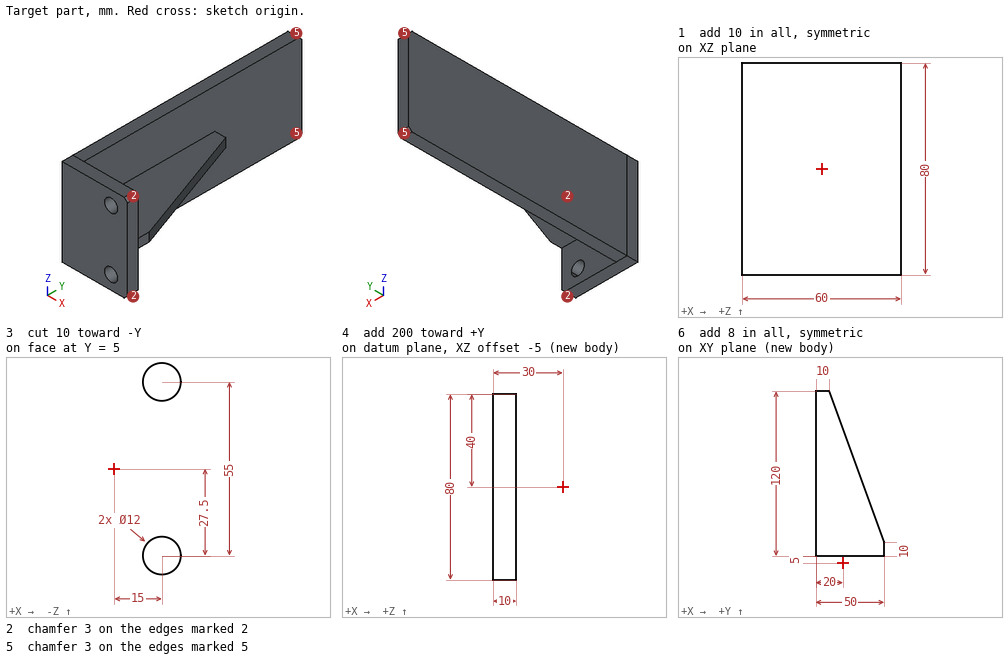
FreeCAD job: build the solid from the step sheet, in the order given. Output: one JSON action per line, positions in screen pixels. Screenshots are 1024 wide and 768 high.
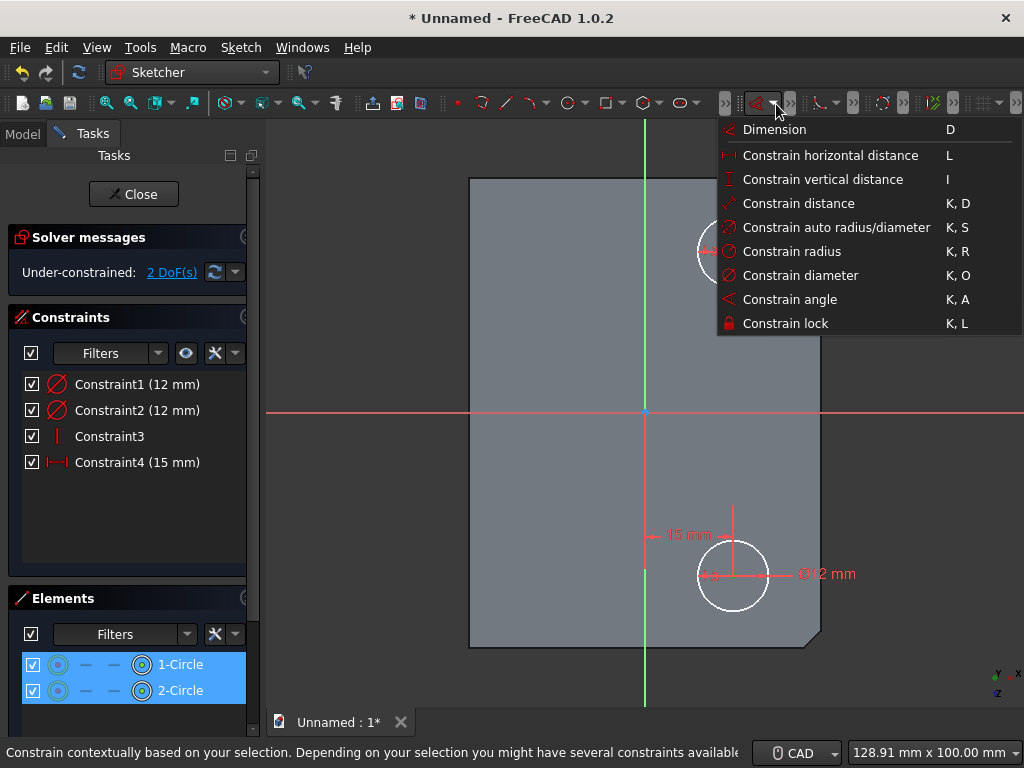
{"action": "left_click", "coordinate": [870, 179]}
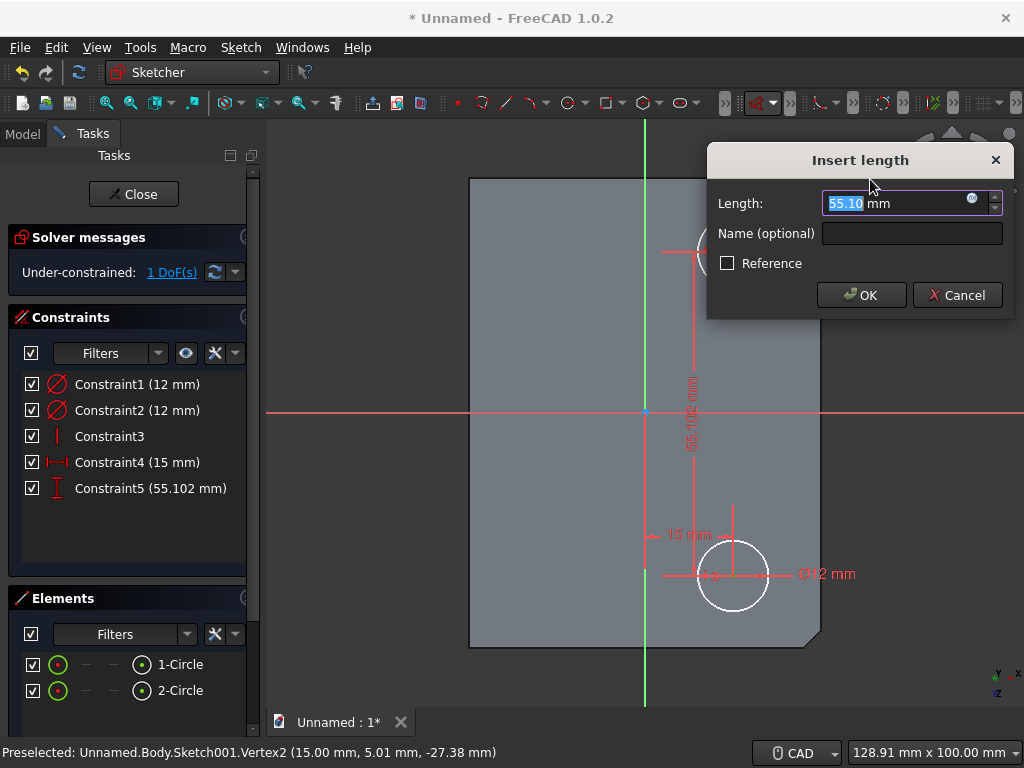
{"action": "type", "text": "55"}
{"action": "key", "text": "Return"}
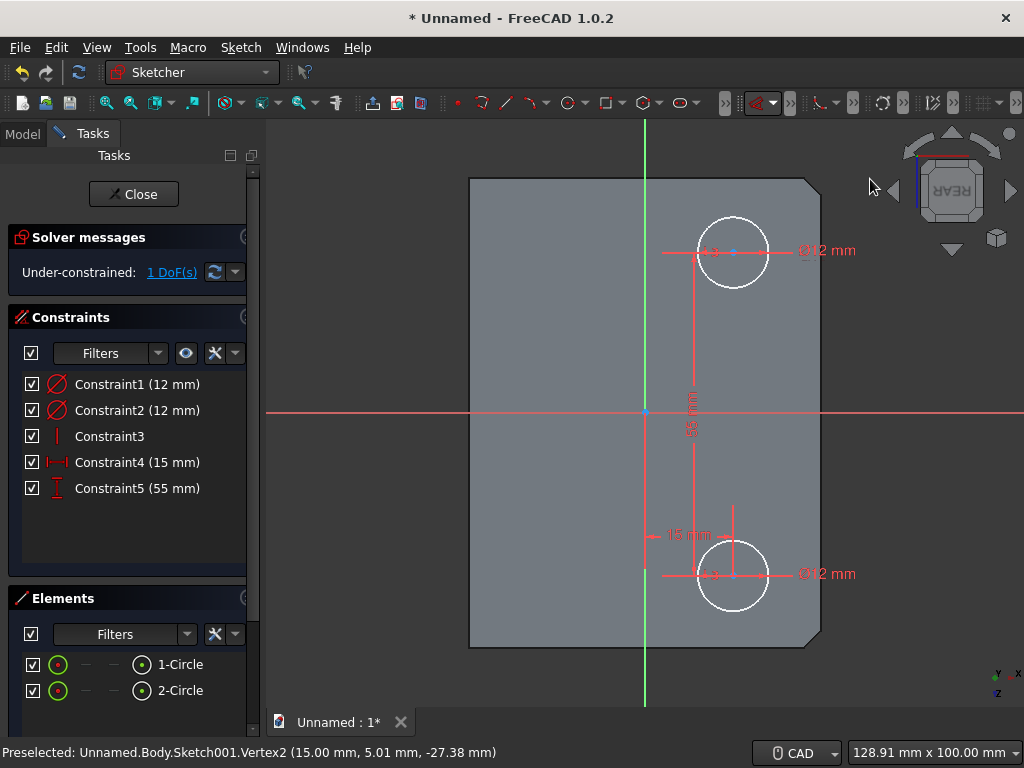
{"action": "left_click", "coordinate": [733, 576]}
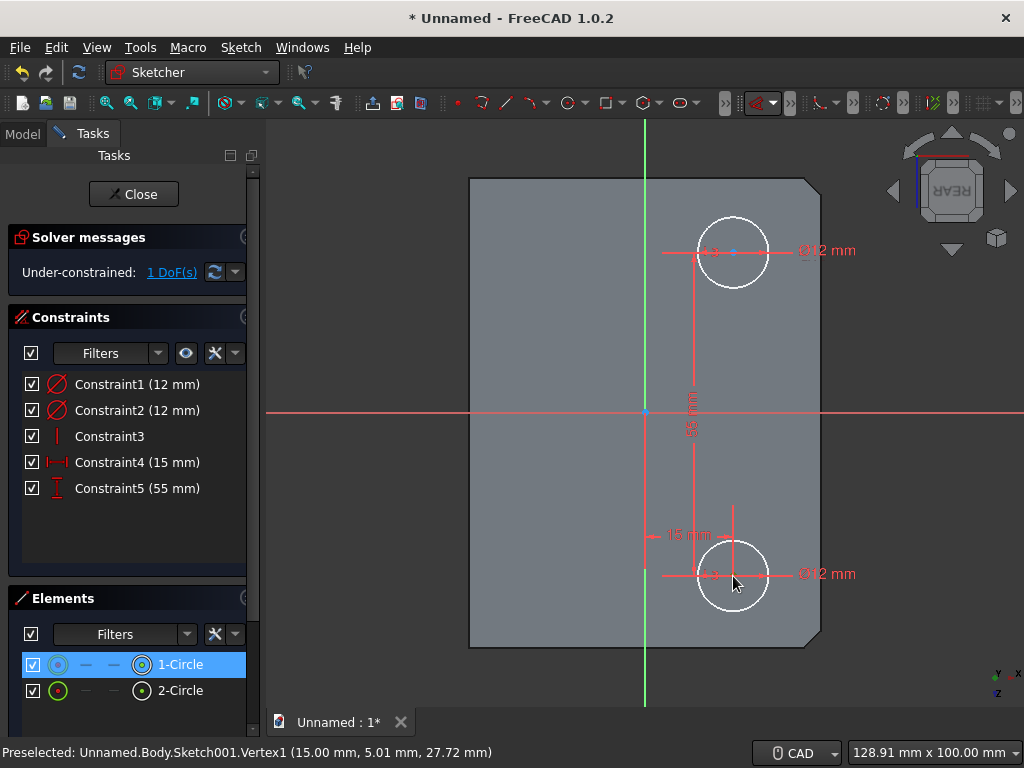
{"action": "key", "text": "i"}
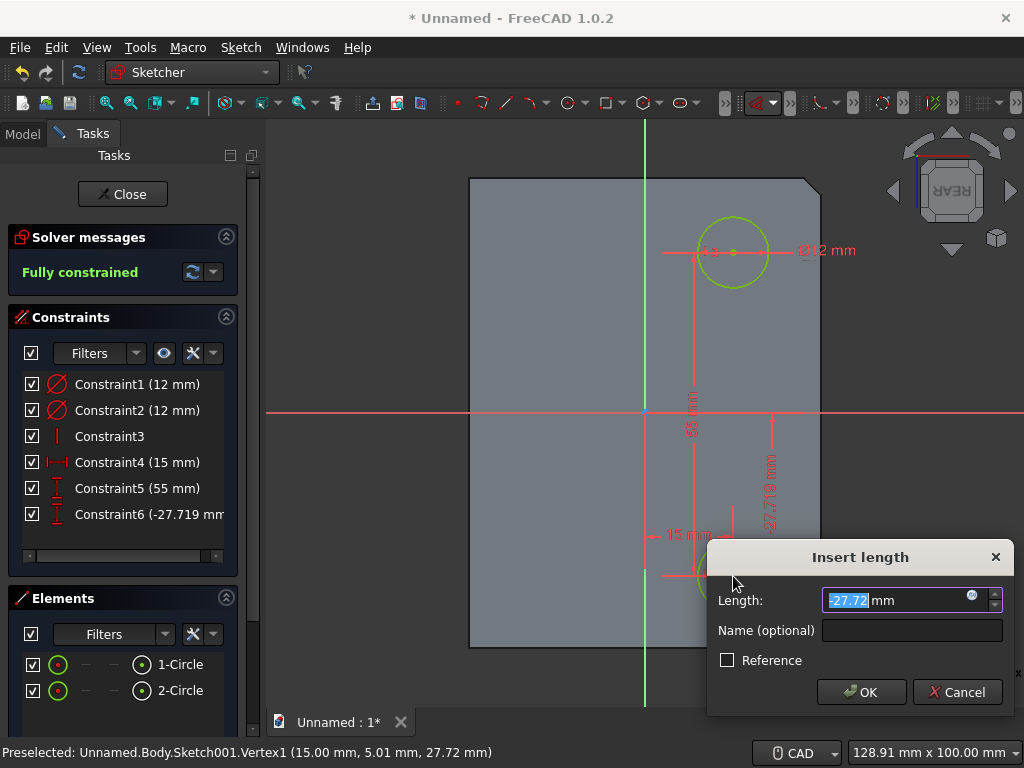
{"action": "type", "text": "-27.5"}
{"action": "key", "text": "Return"}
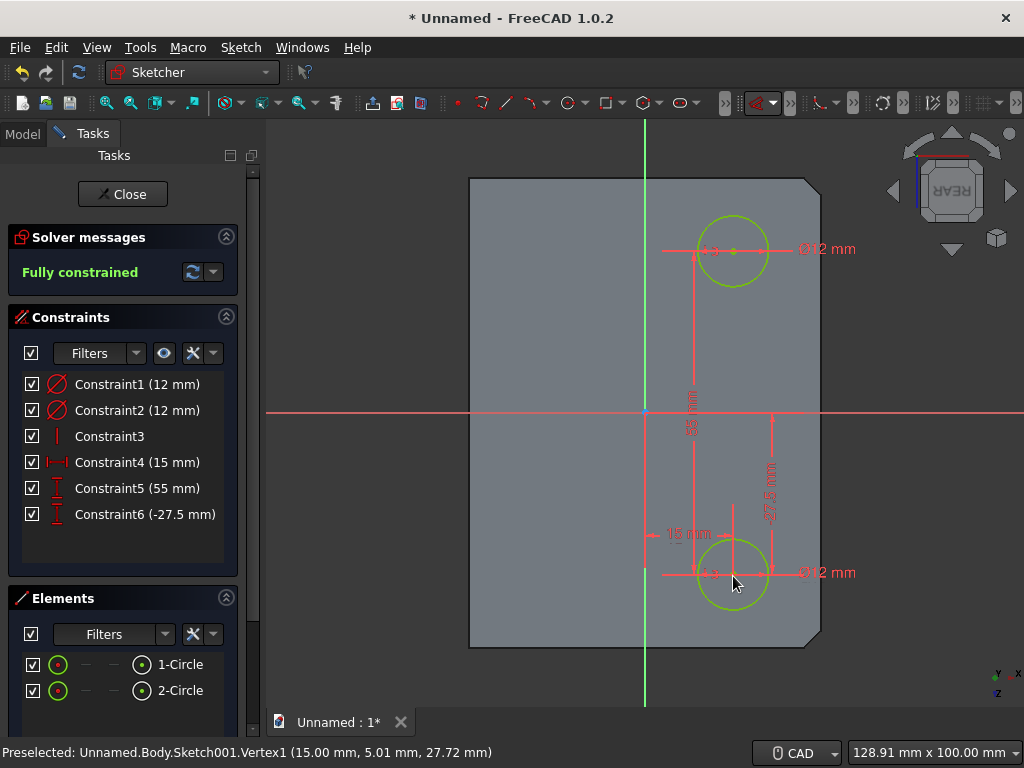
{"action": "left_click", "coordinate": [123, 194]}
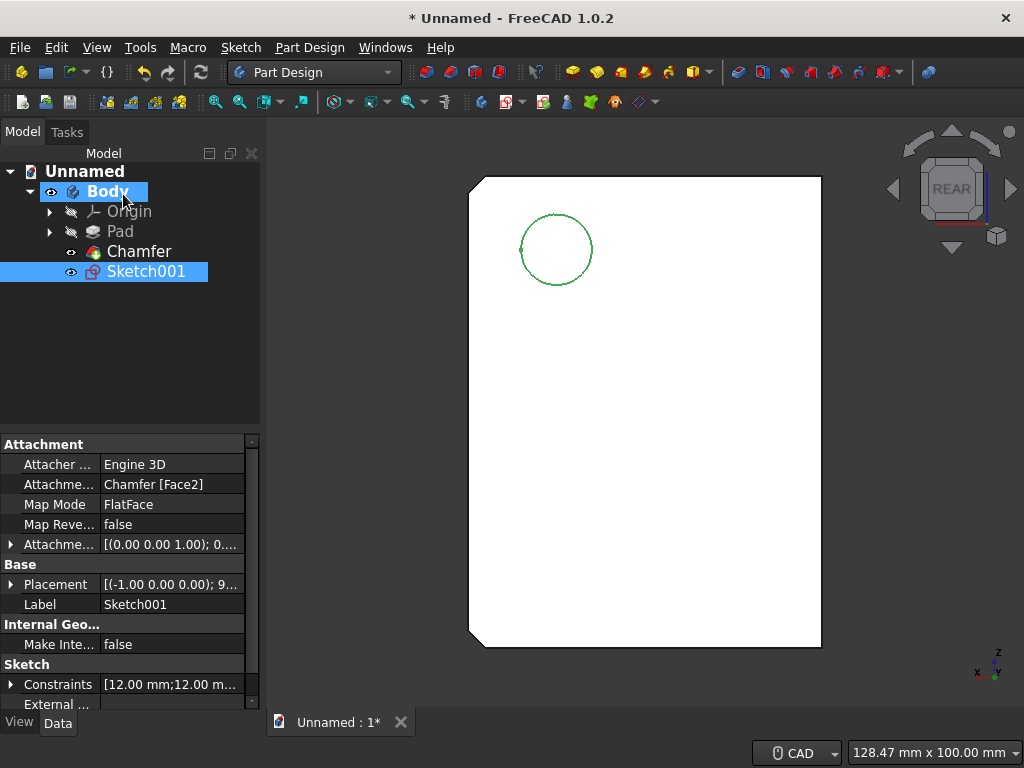
{"action": "left_click", "coordinate": [740, 72]}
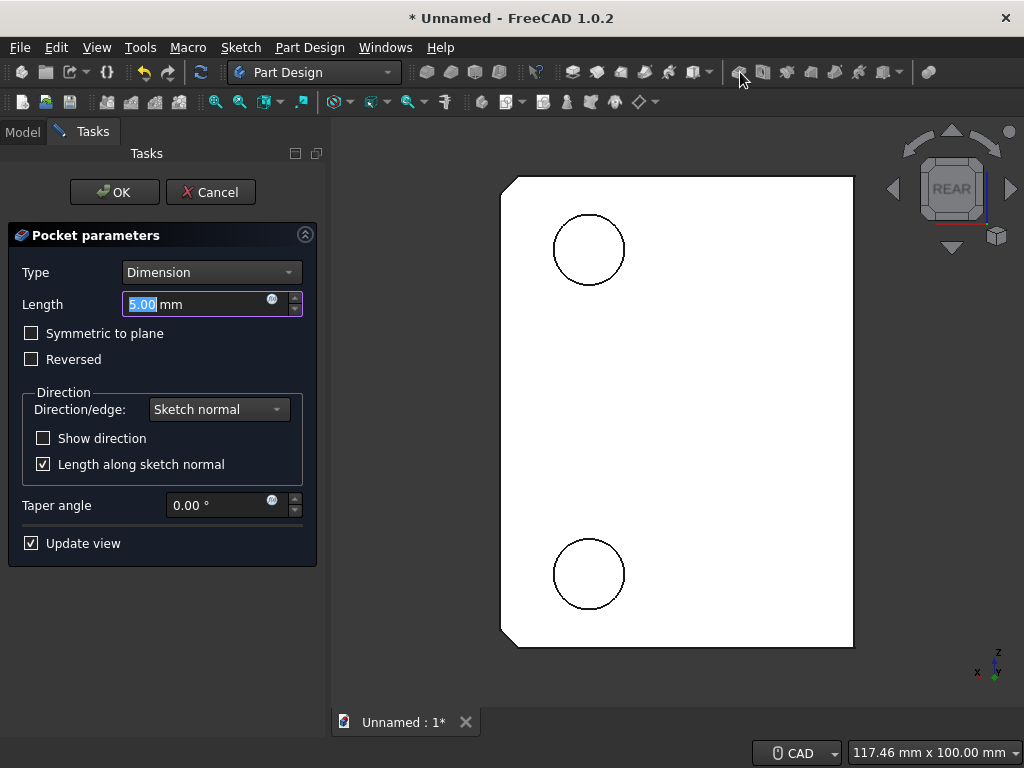
{"action": "type", "text": "10"}
{"action": "key", "text": "Tab"}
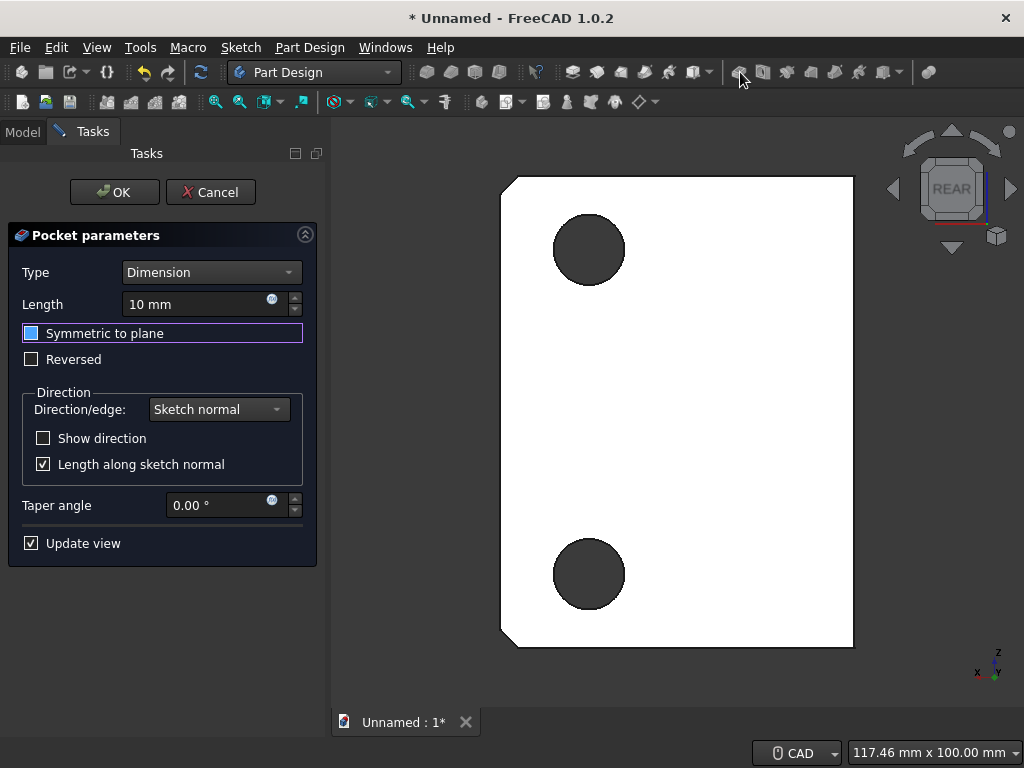
{"action": "left_click", "coordinate": [115, 192]}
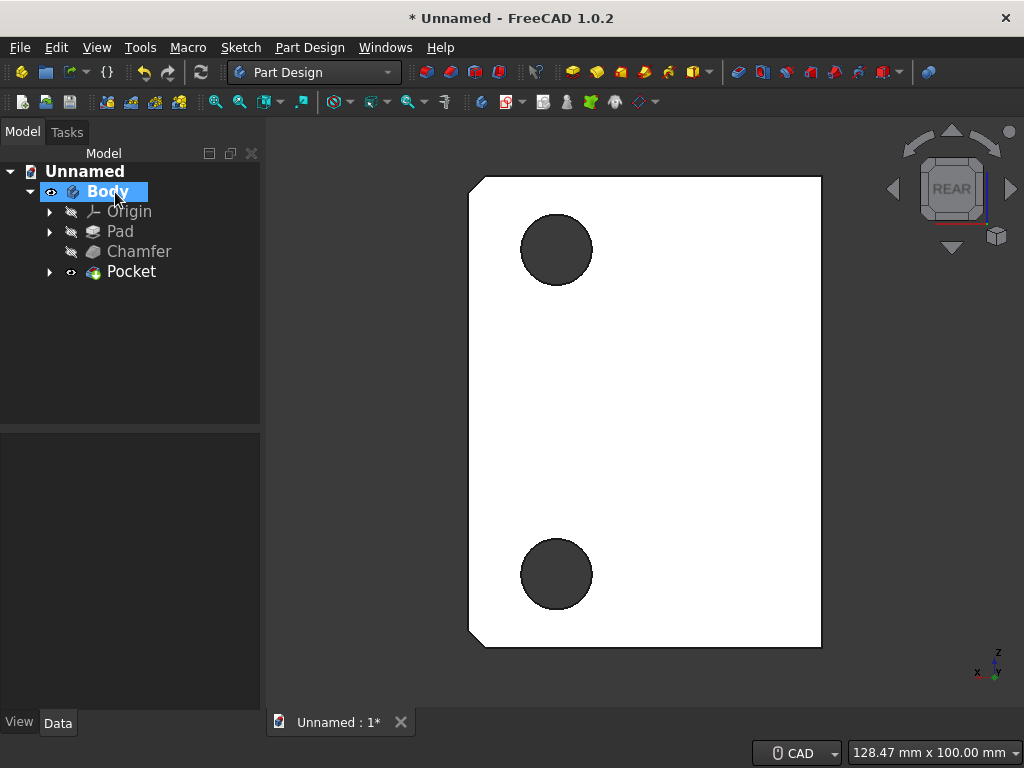
{"action": "left_click", "coordinate": [482, 102]}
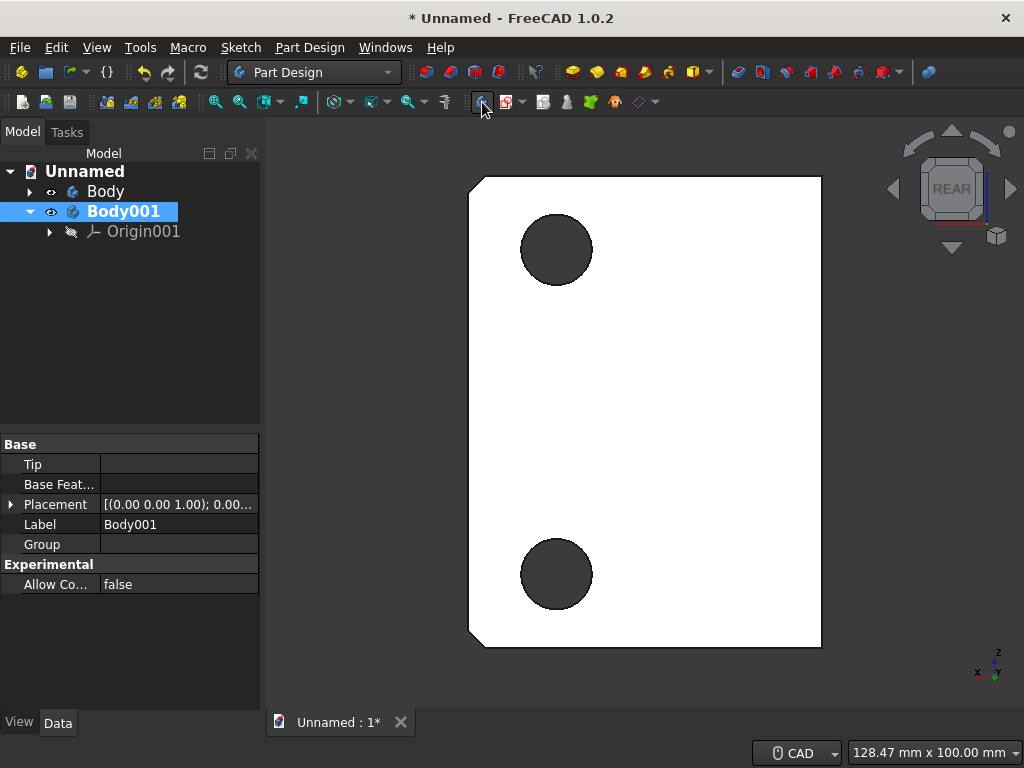
{"action": "left_click", "coordinate": [50, 232]}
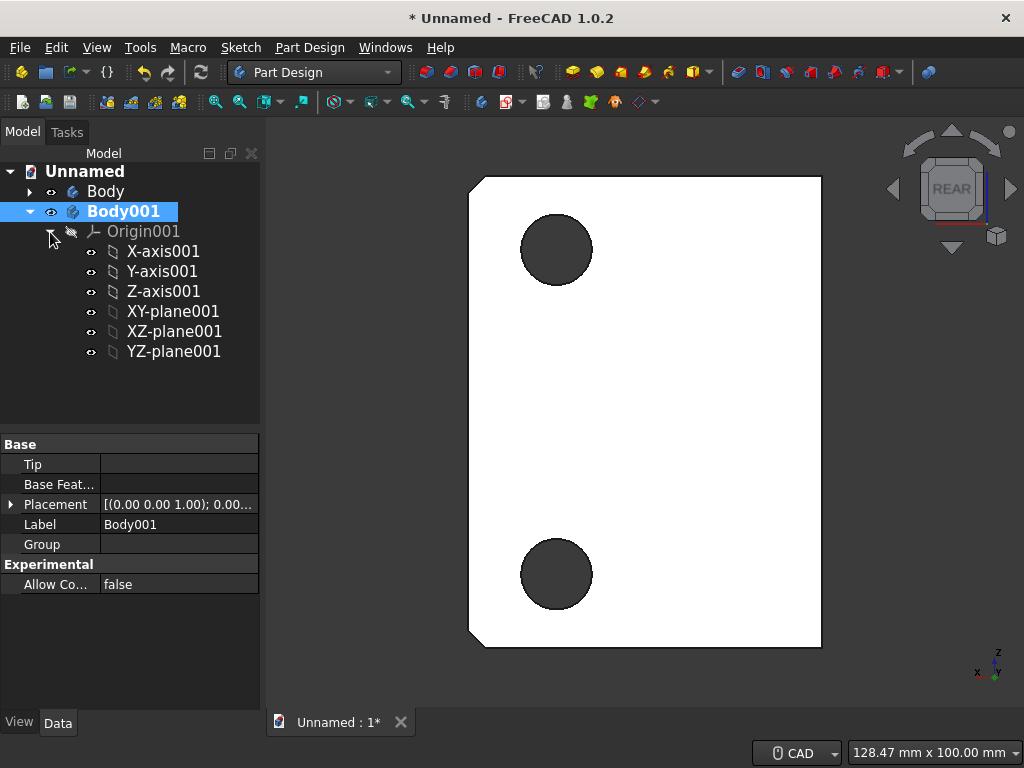
{"action": "left_click", "coordinate": [136, 332]}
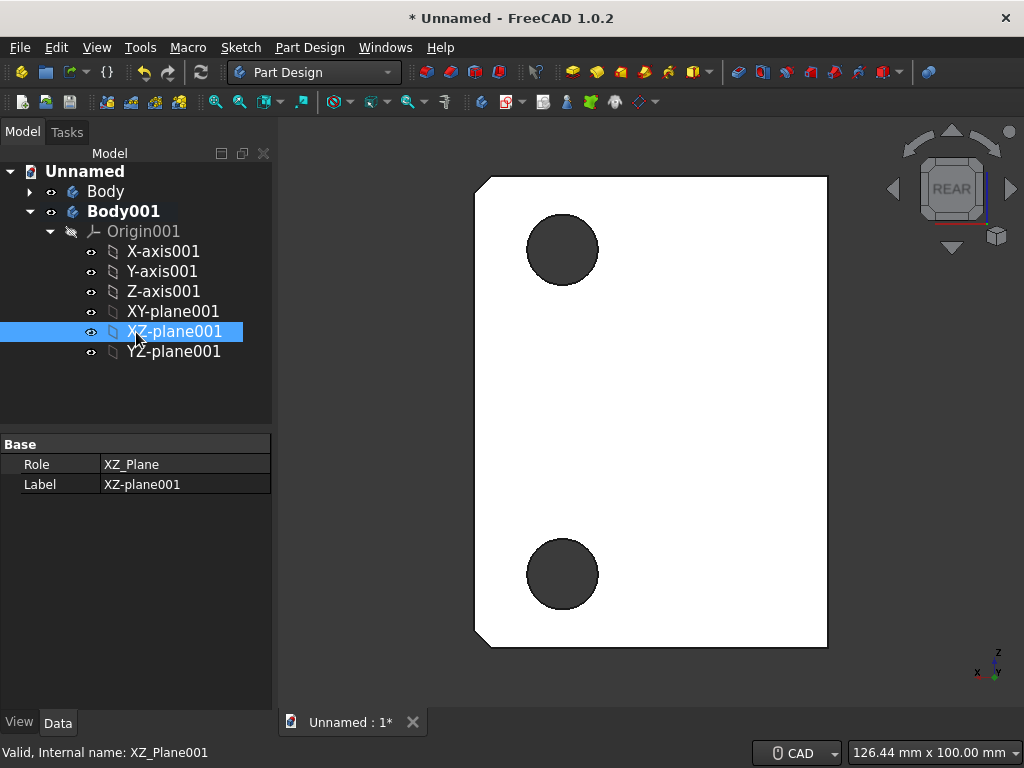
{"action": "left_click", "coordinate": [640, 102]}